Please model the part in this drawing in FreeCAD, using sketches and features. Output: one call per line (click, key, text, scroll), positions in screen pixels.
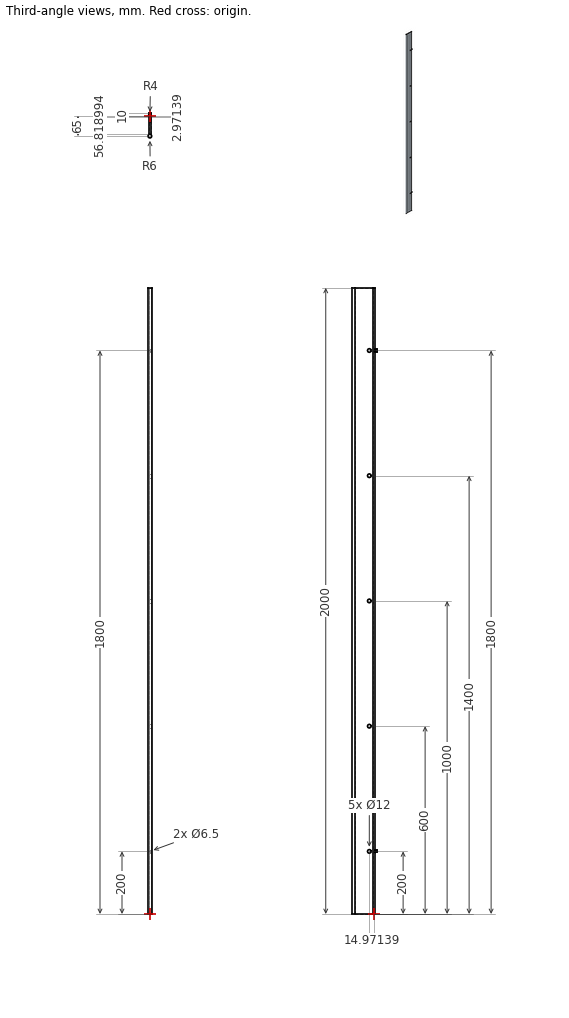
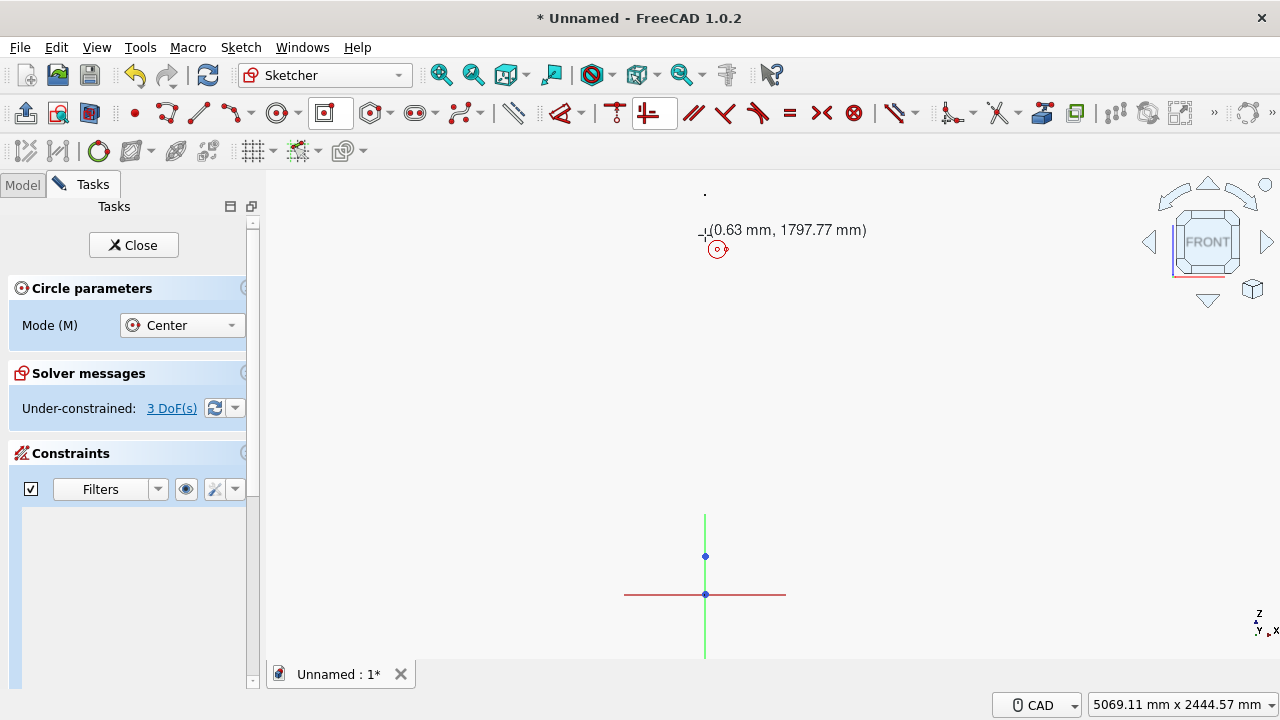
click(705, 235)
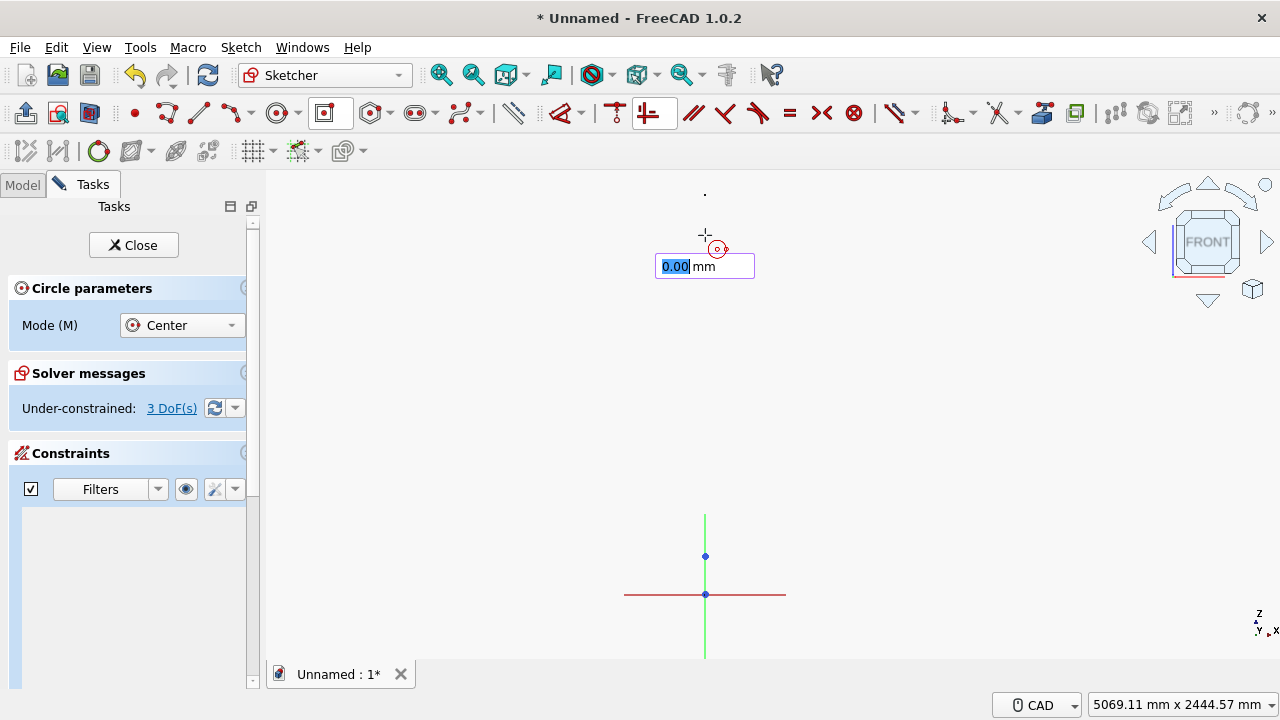
scroll(706, 234, up, 17)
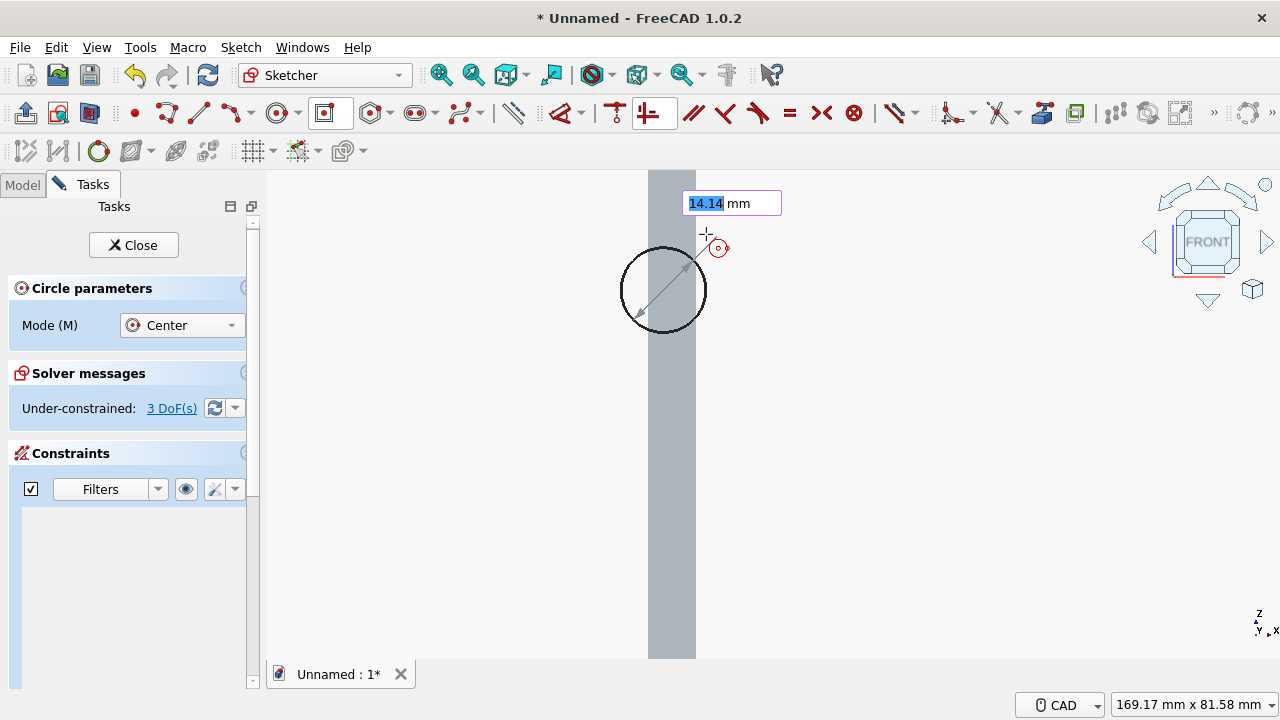
click(691, 245)
key(Escape)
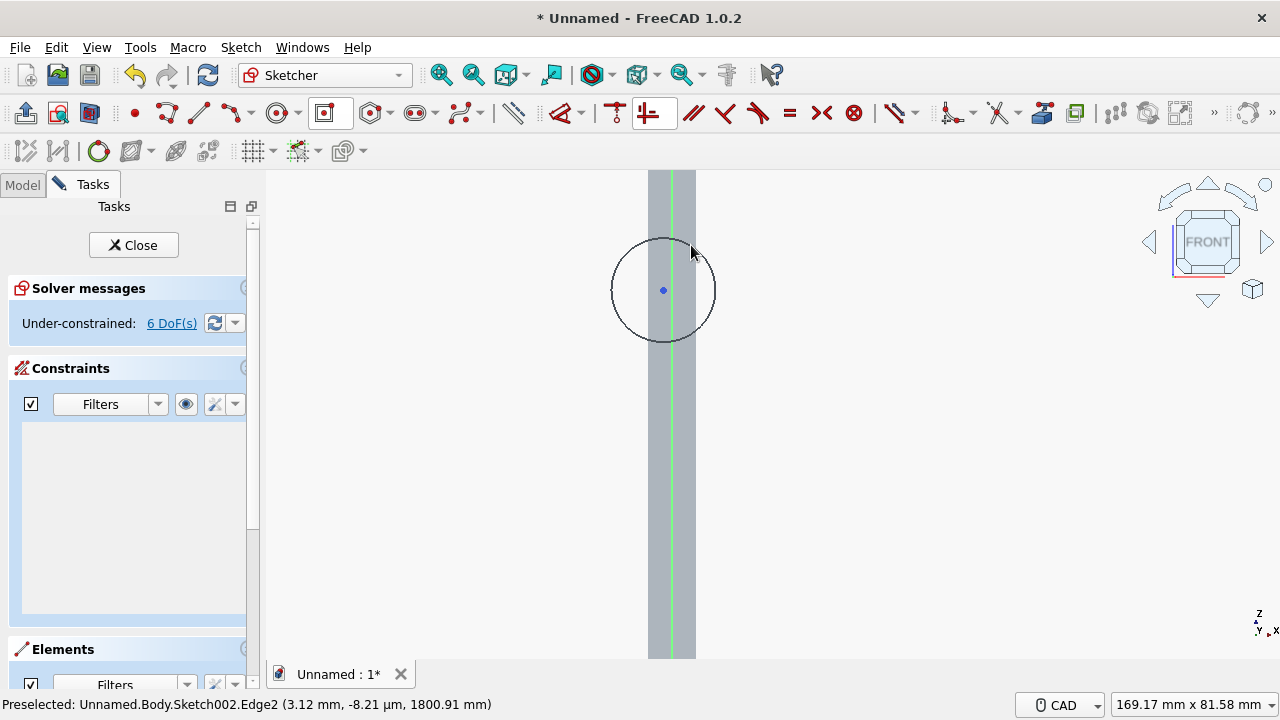
scroll(706, 234, down, 17)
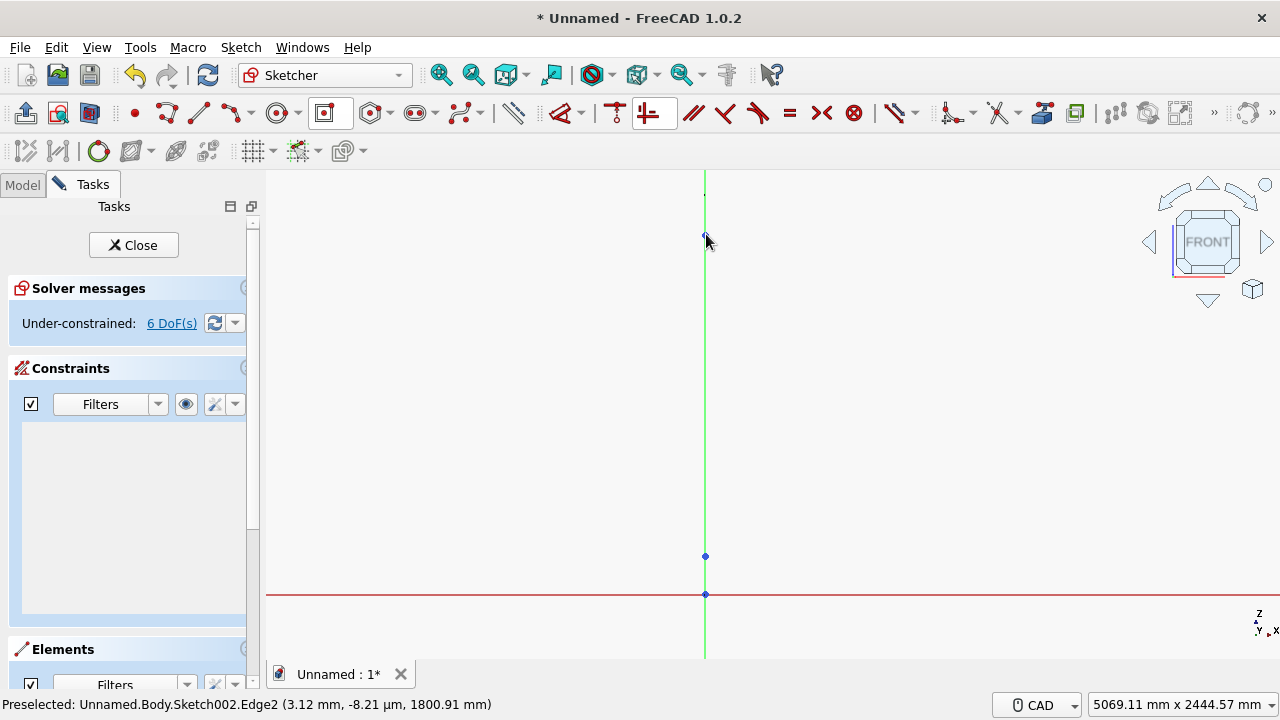
scroll(706, 555, up, 13)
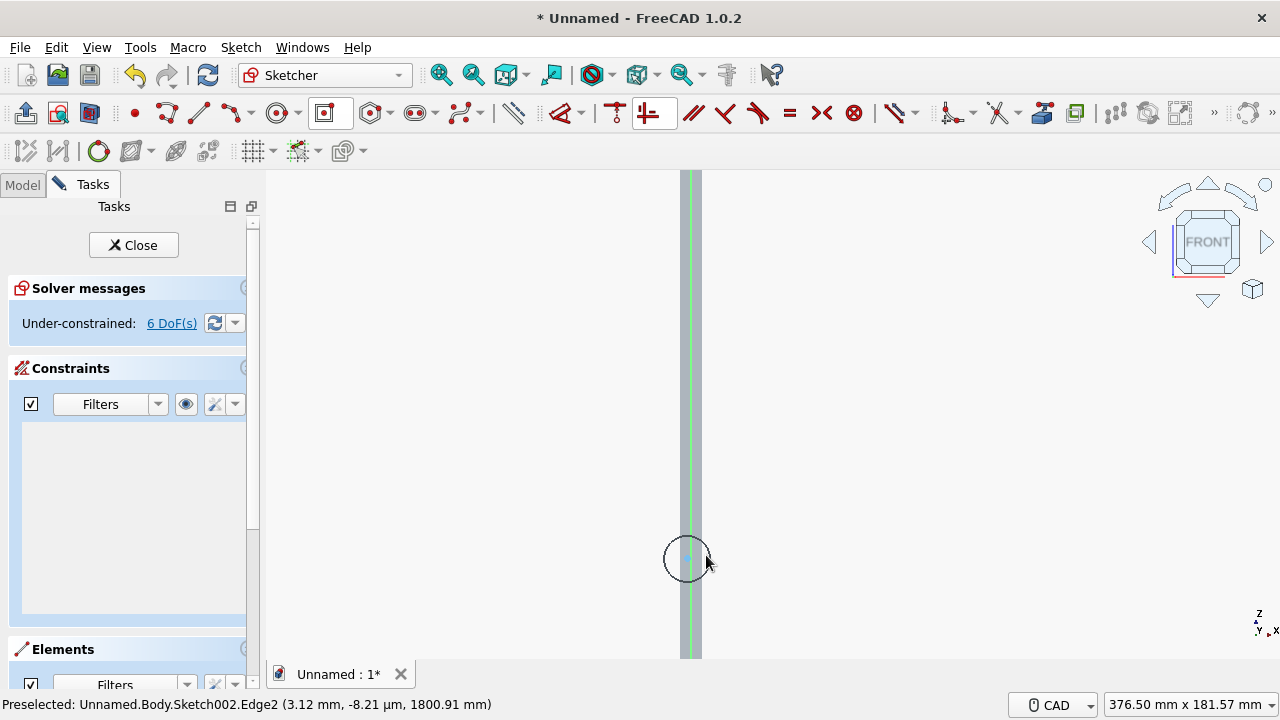
click(703, 543)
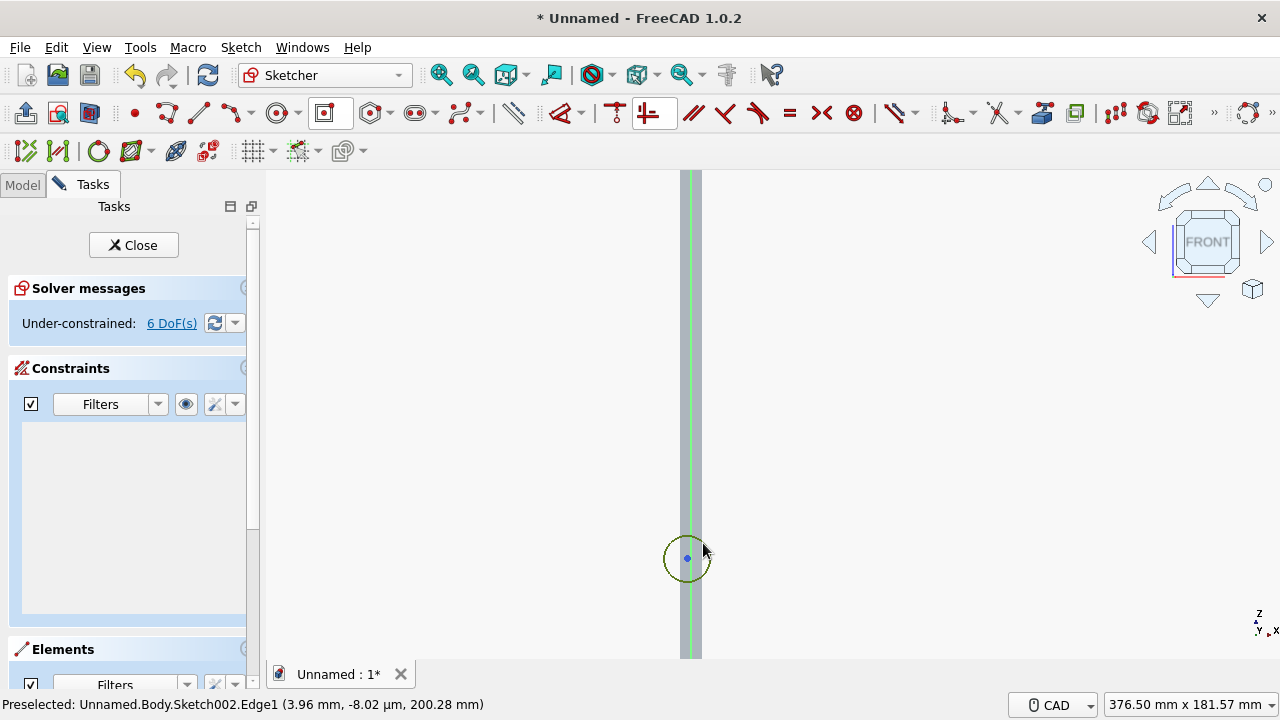
scroll(705, 529, down, 14)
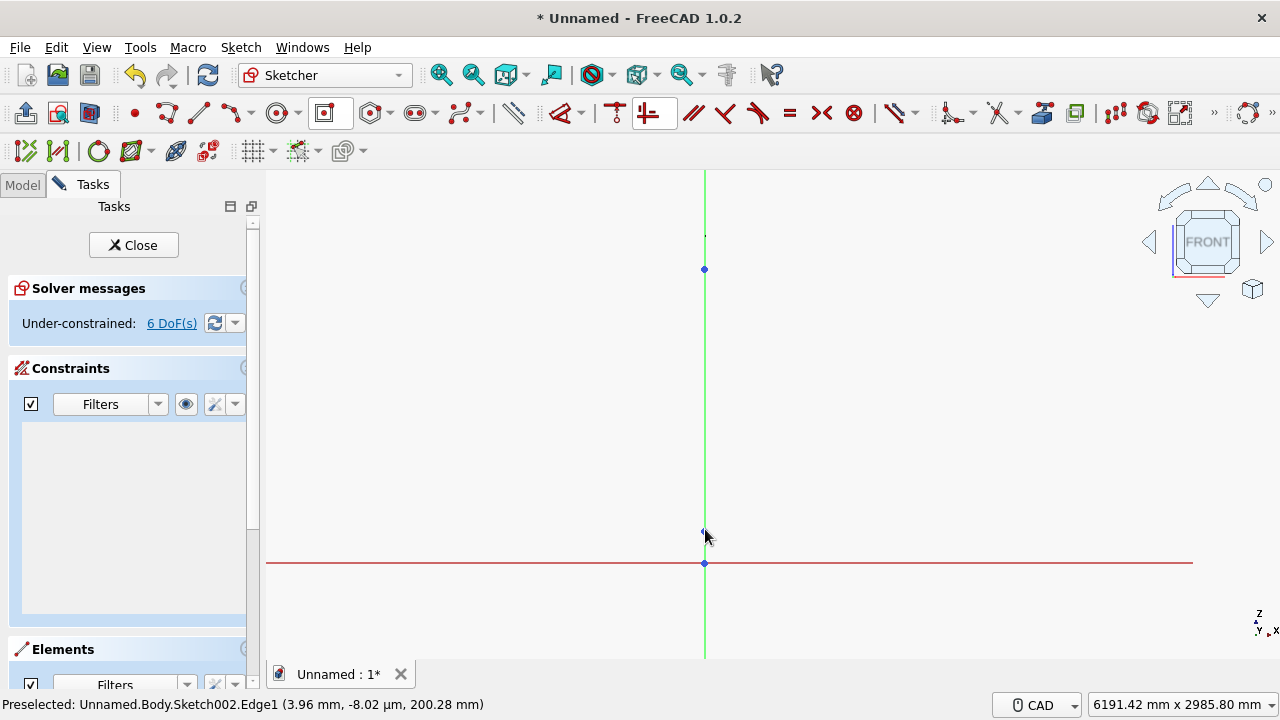
scroll(705, 268, up, 14)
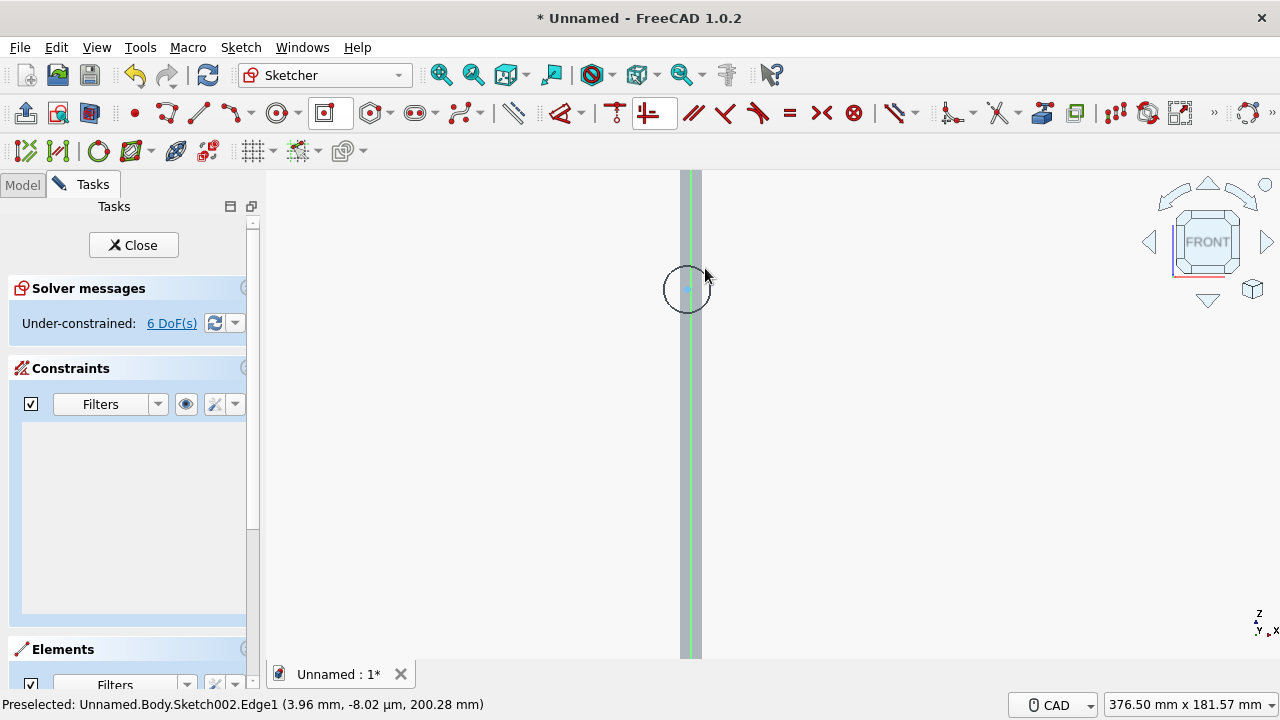
click(704, 273)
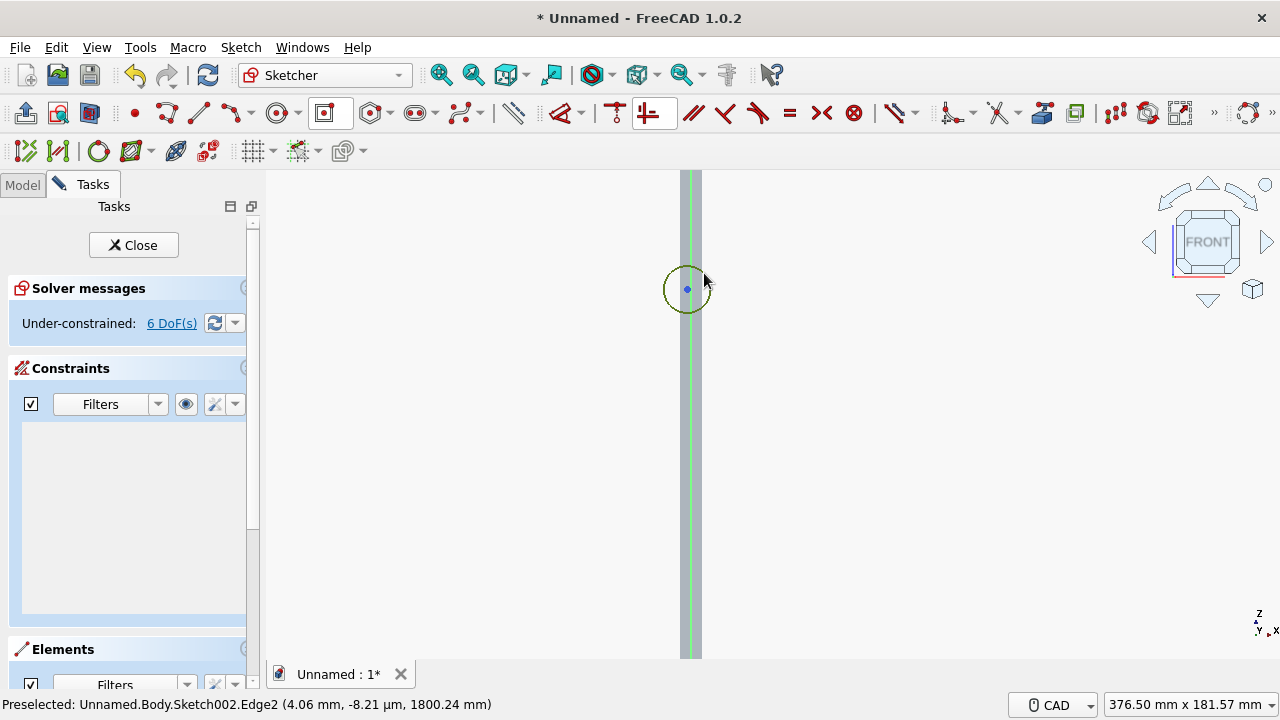
key(e)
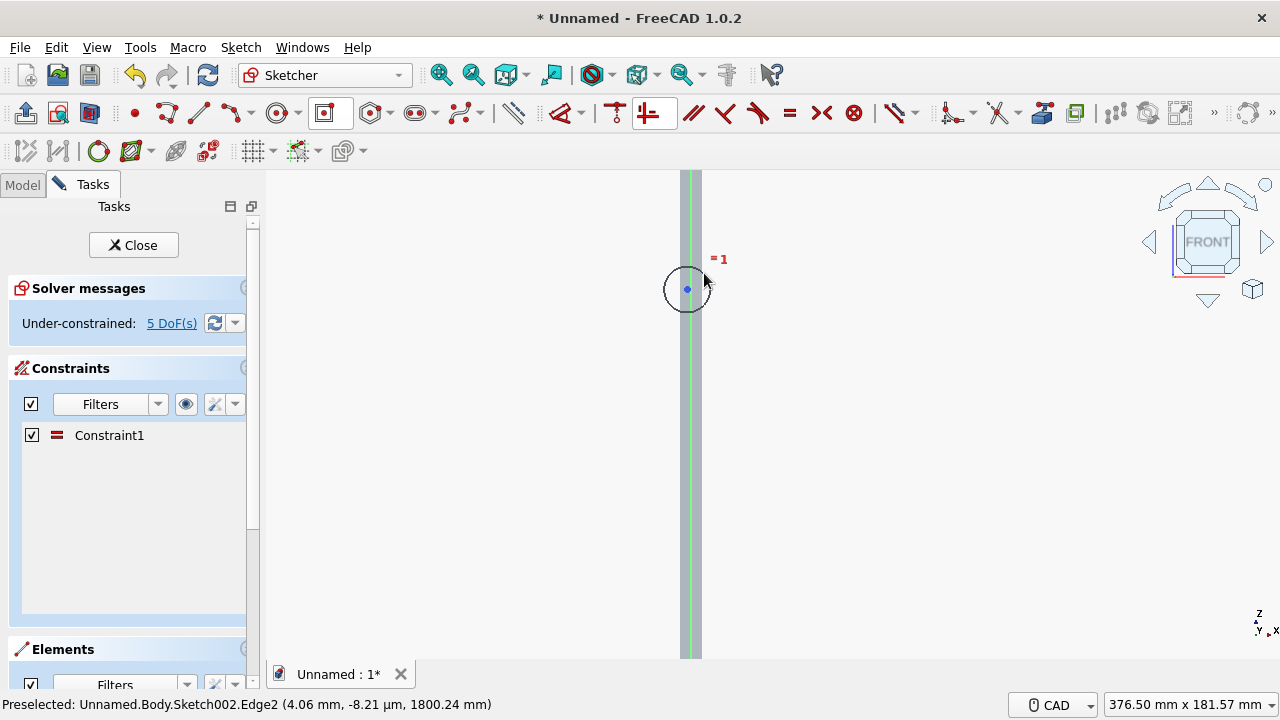
scroll(705, 267, down, 14)